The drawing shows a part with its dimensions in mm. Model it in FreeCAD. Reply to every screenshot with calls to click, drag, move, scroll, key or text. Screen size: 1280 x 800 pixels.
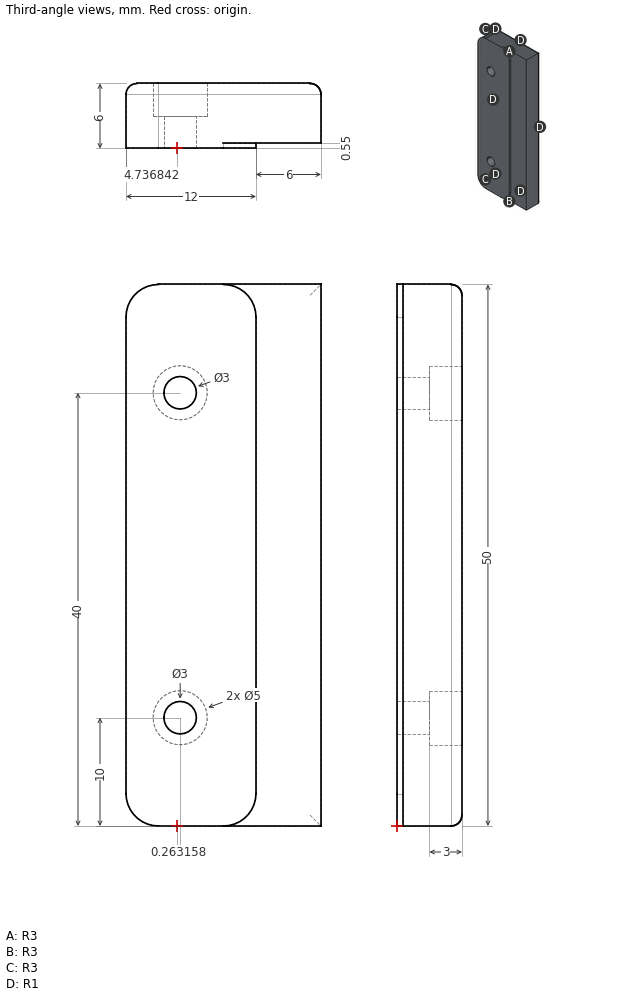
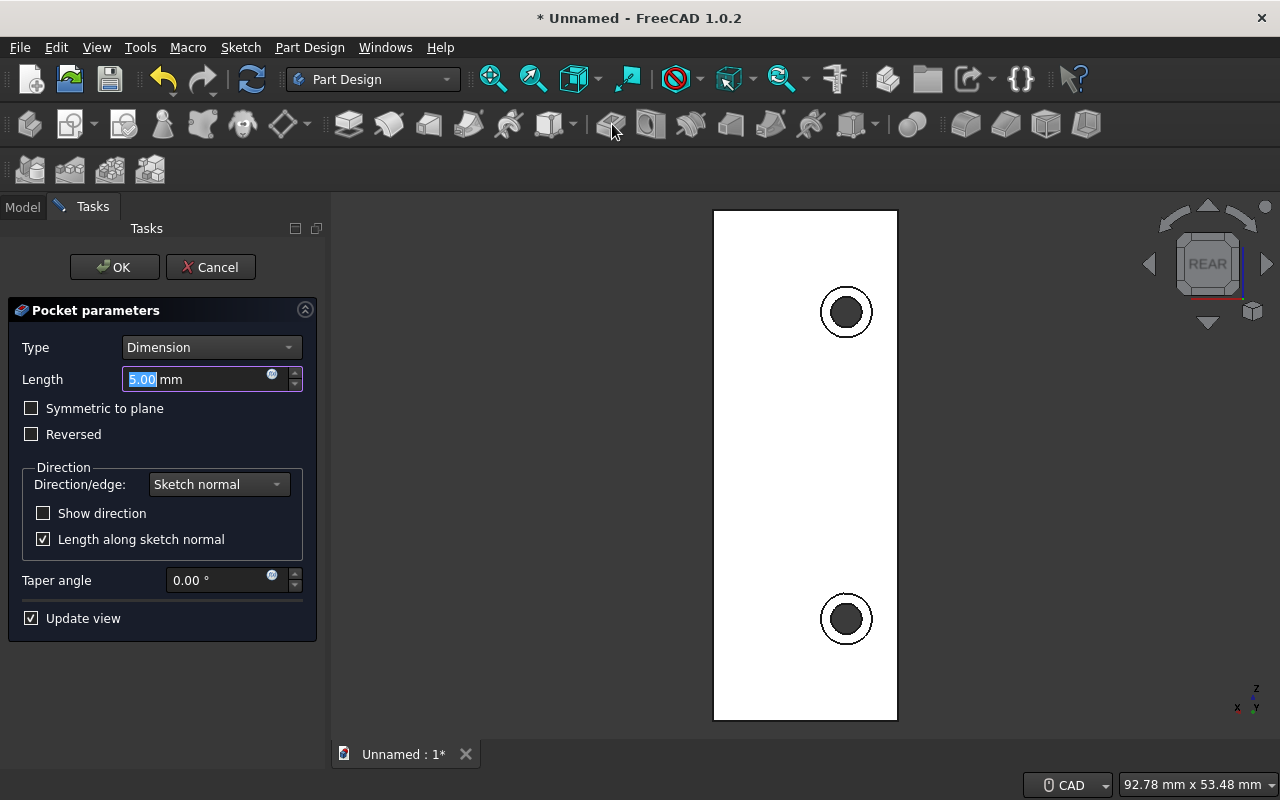
click(212, 348)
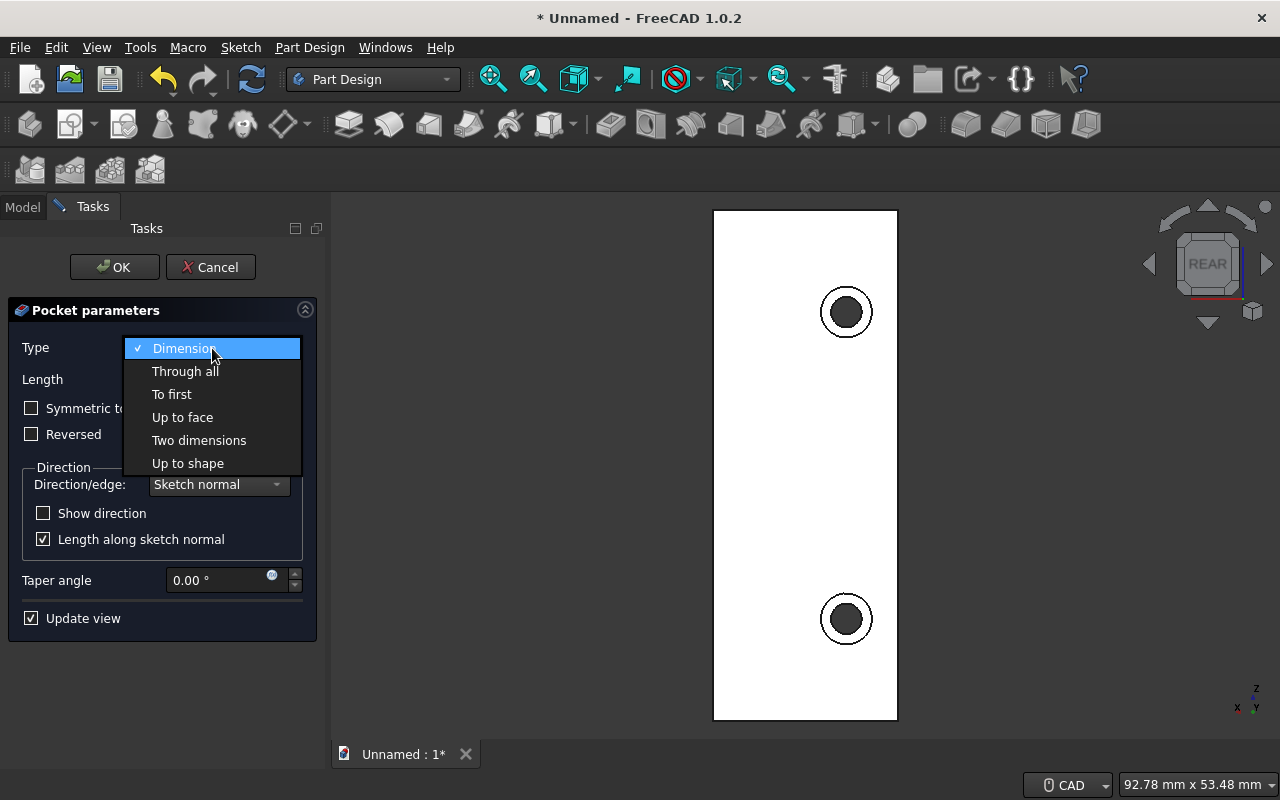
click(212, 372)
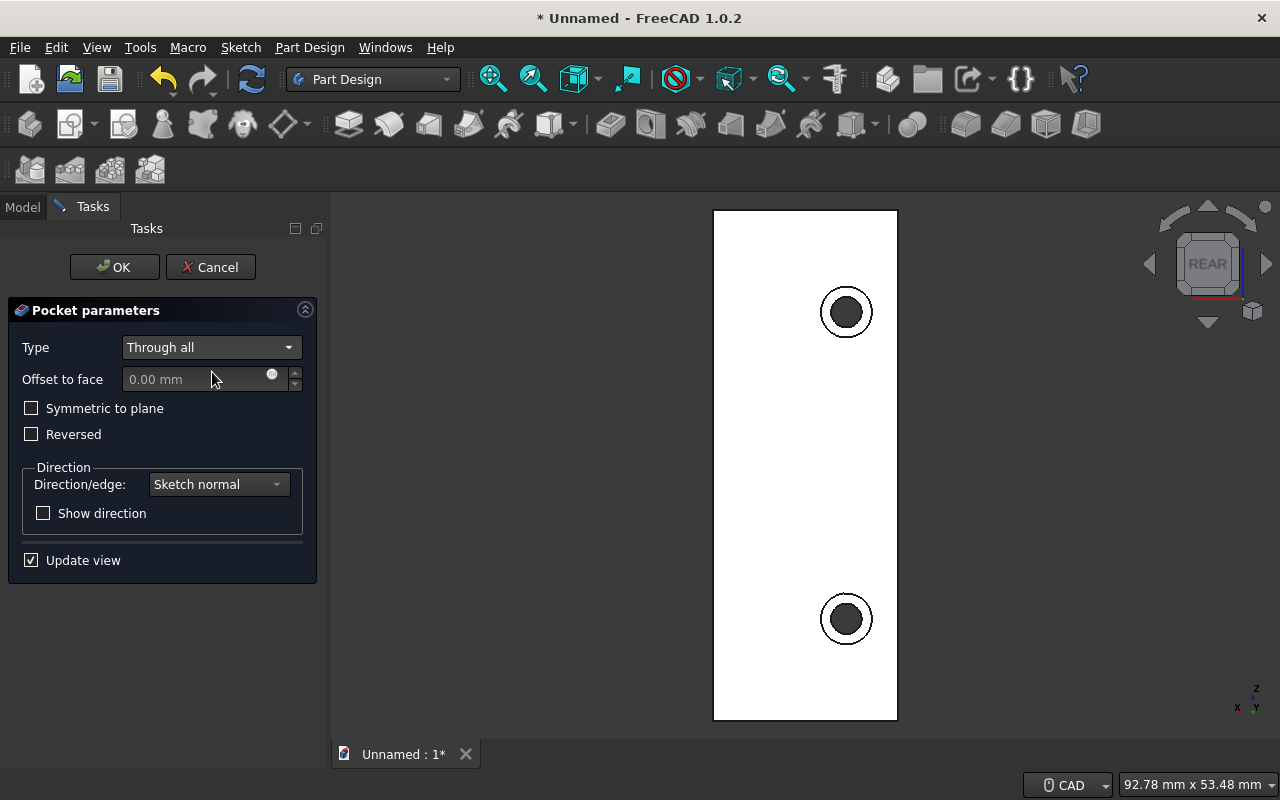
click(115, 267)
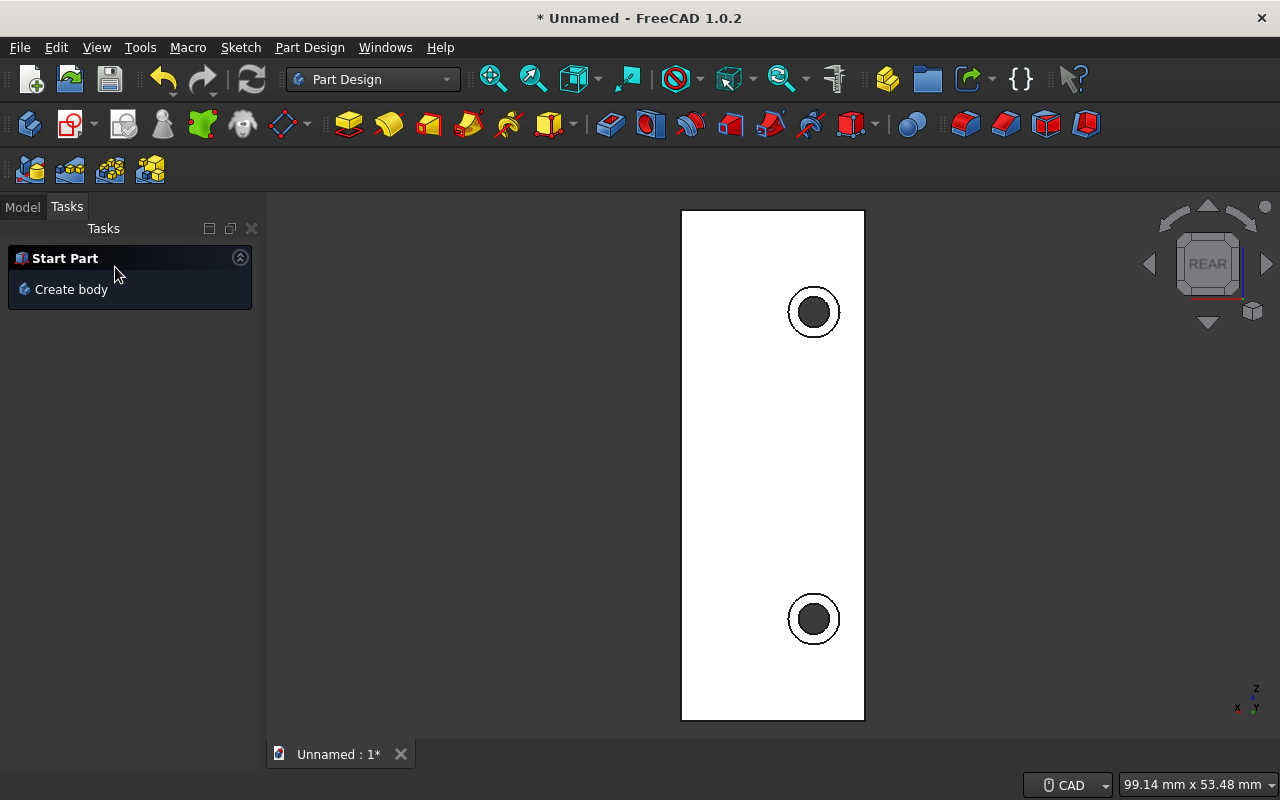
key(0)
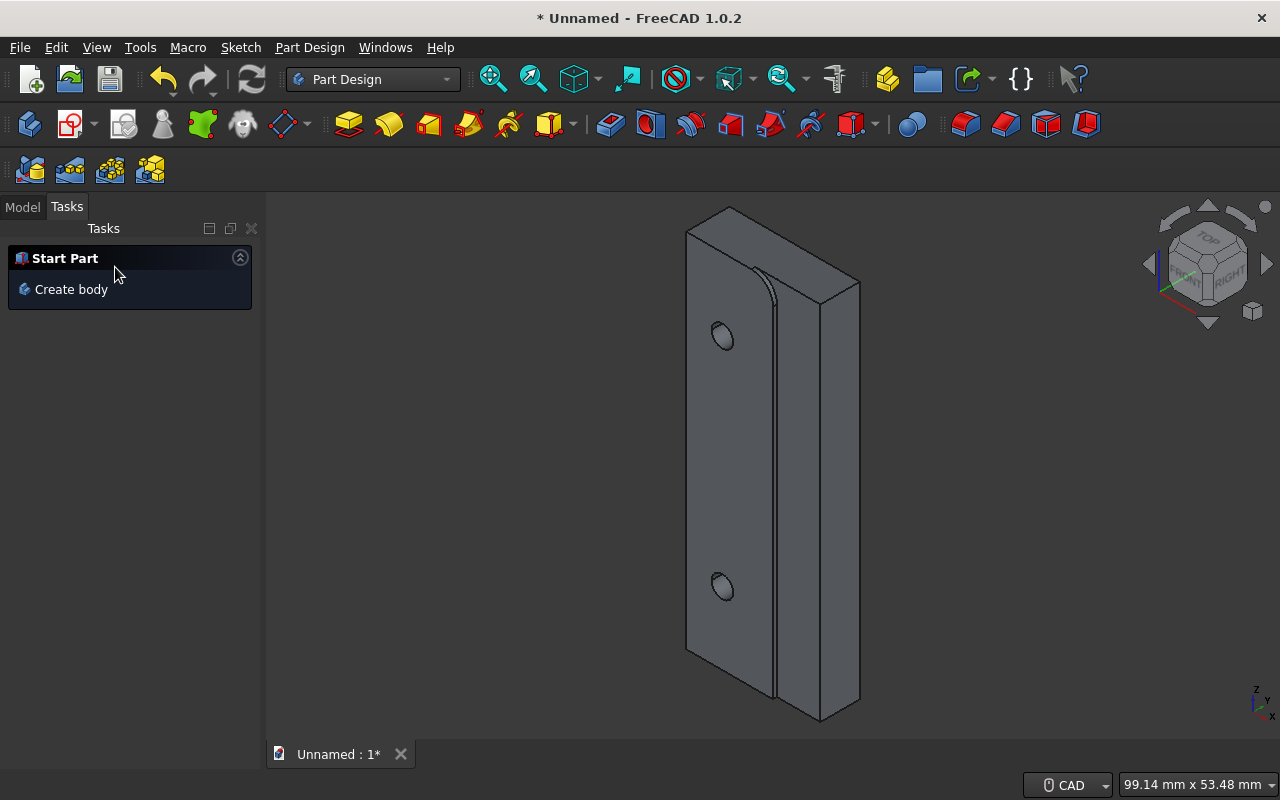
scroll(775, 697, up, 10)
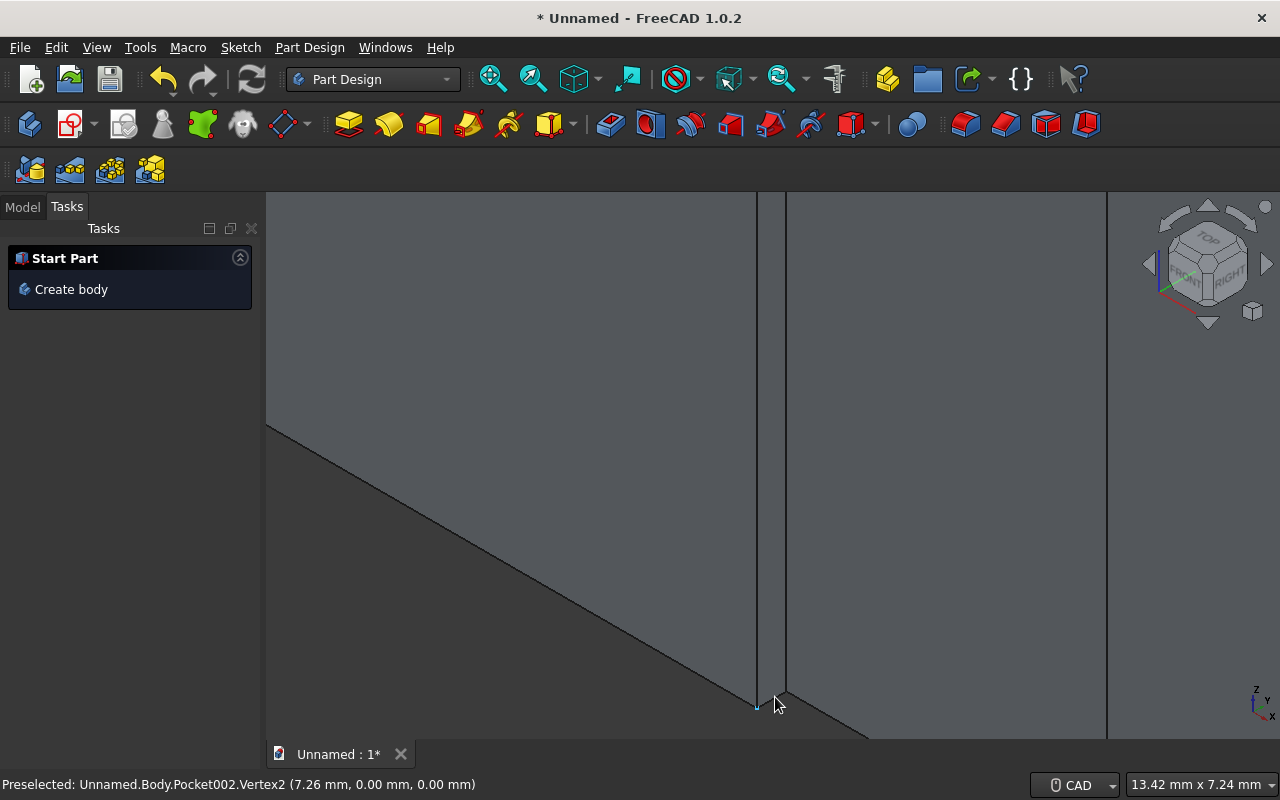
click(494, 80)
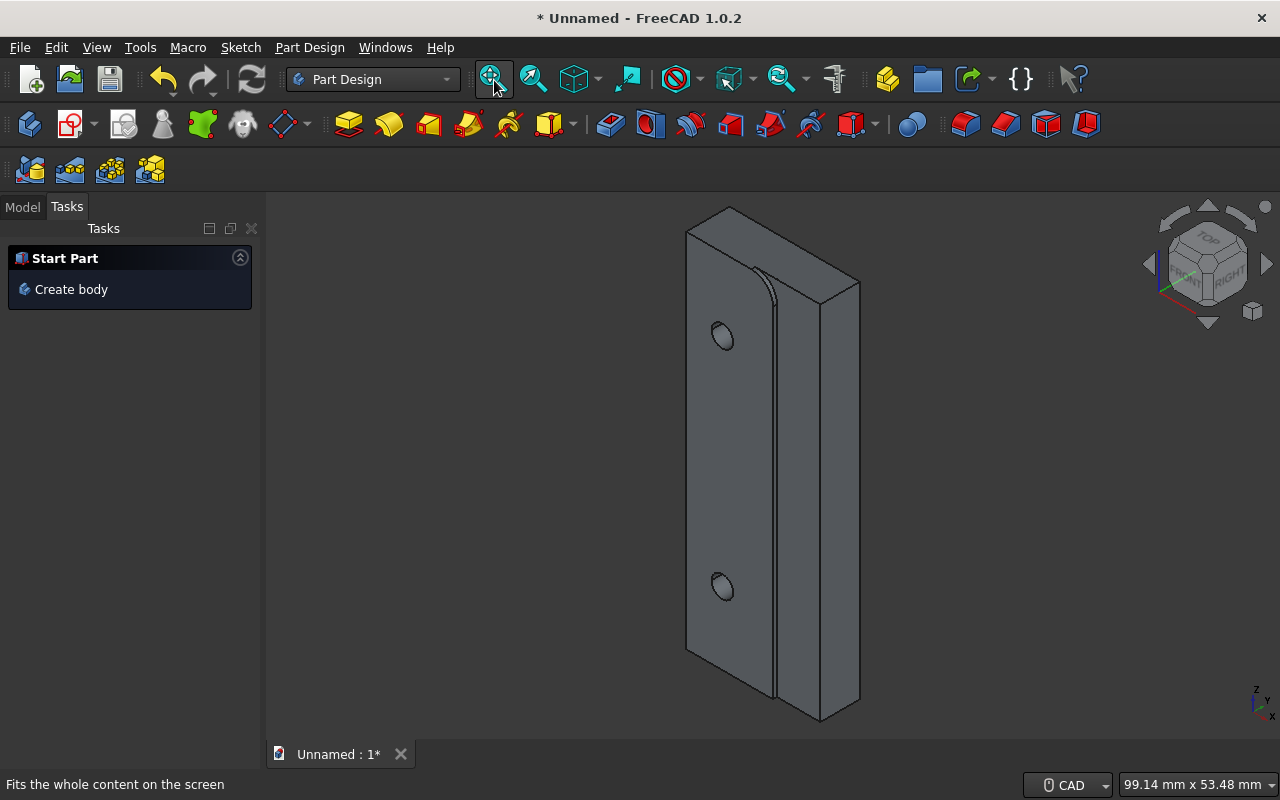
key(2)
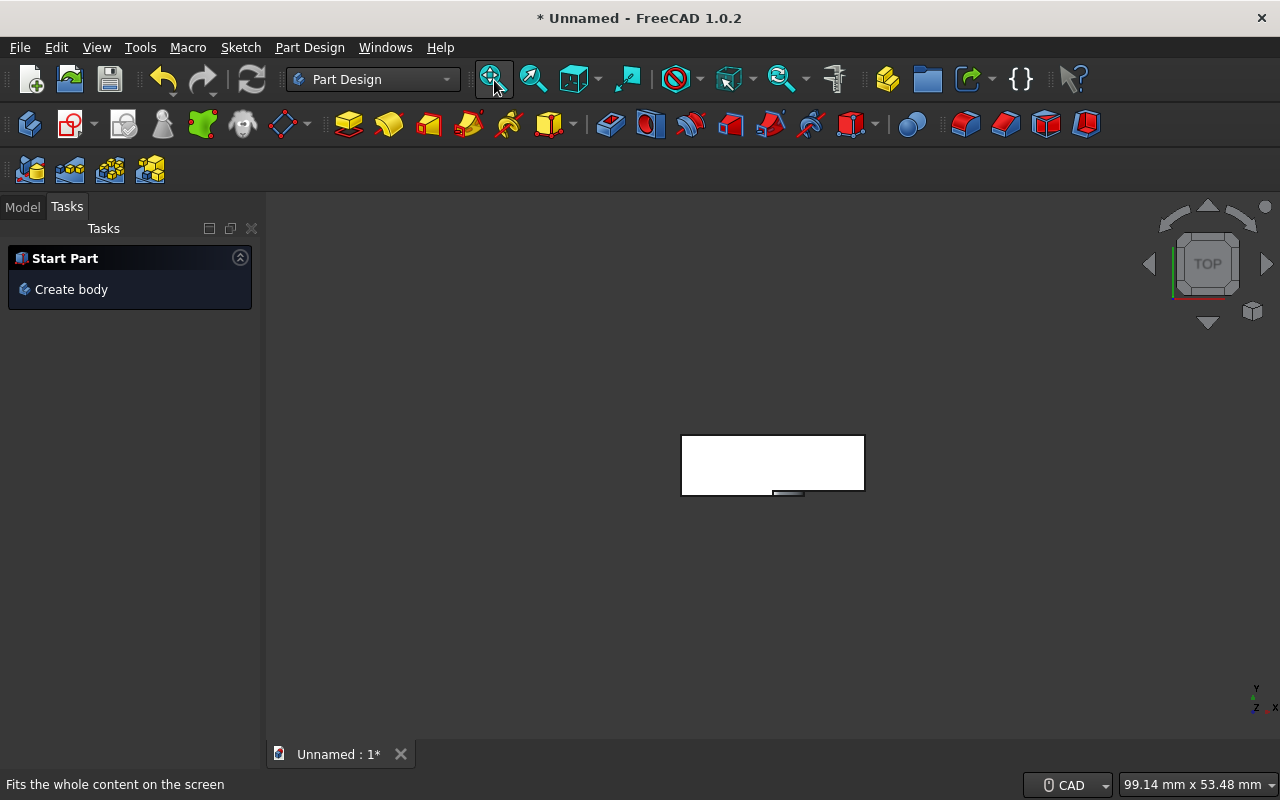
click(494, 80)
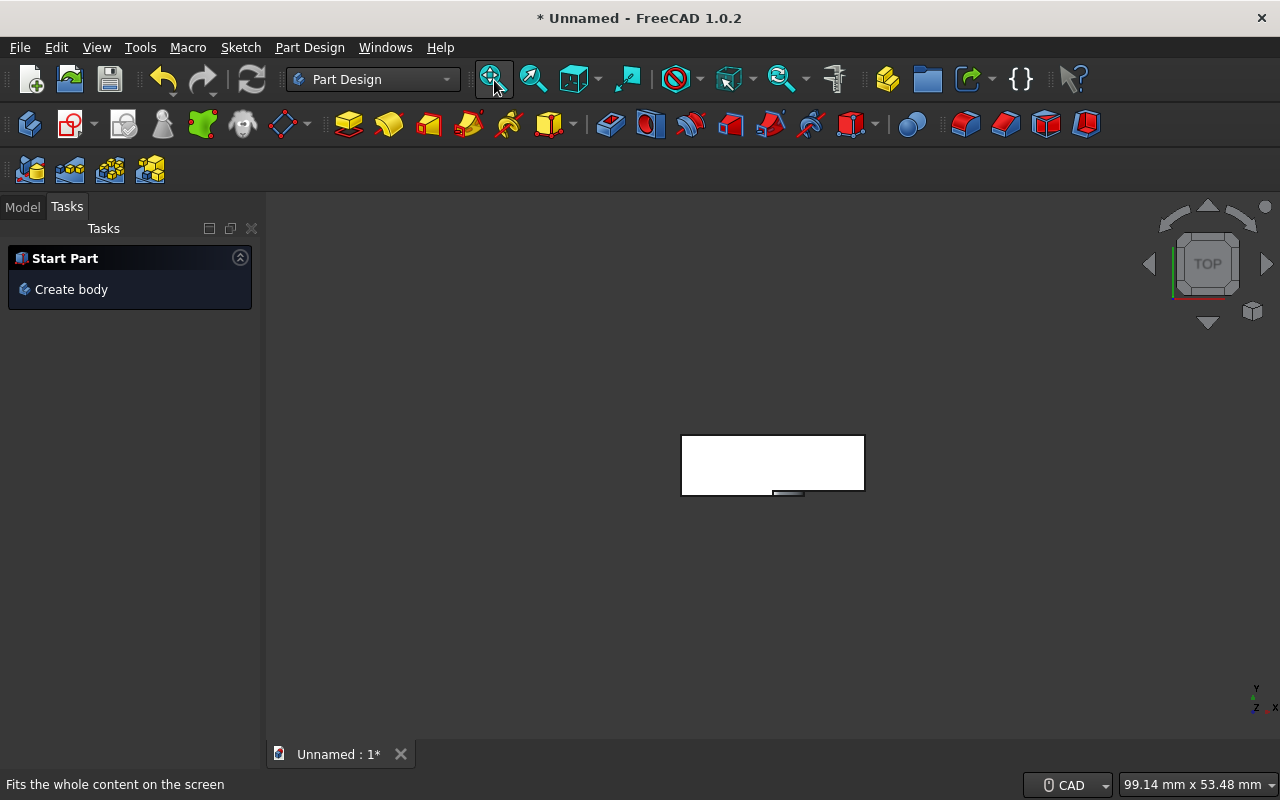
scroll(804, 492, up, 10)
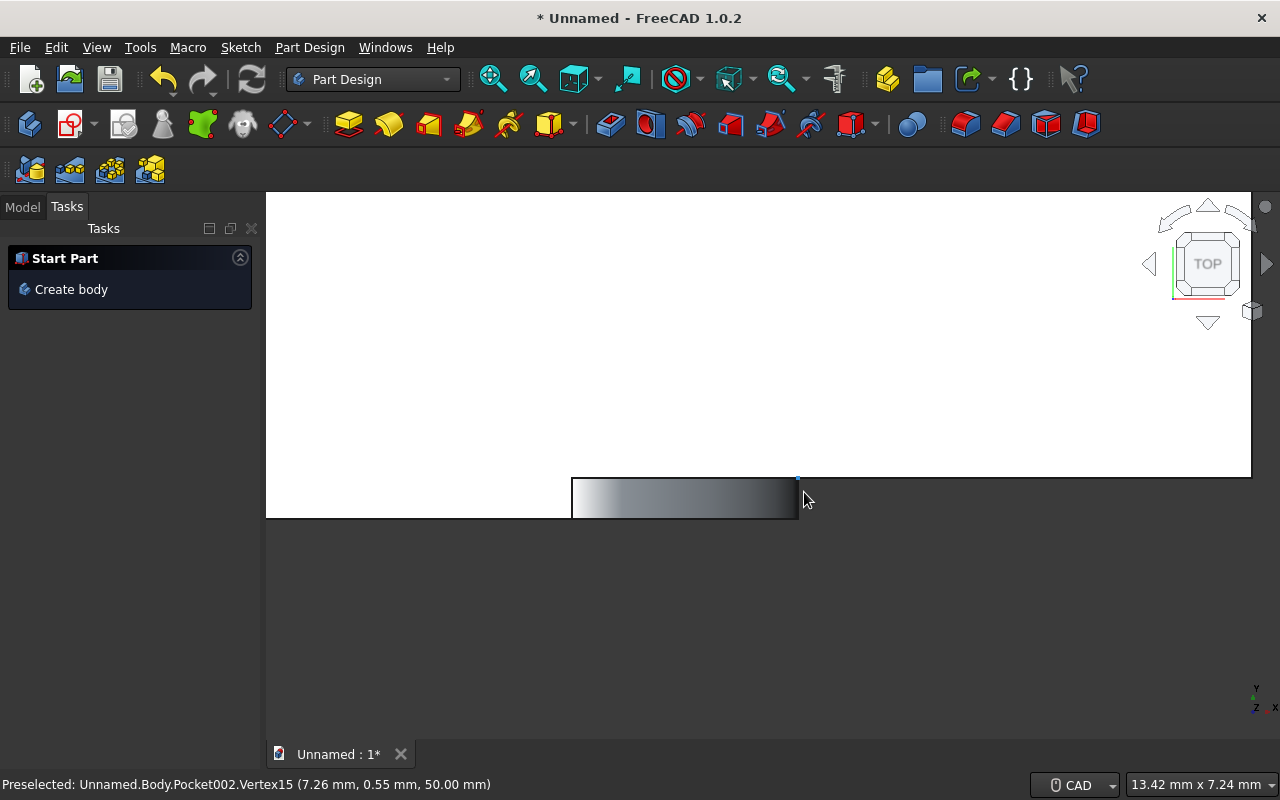
key(v)
key(f)